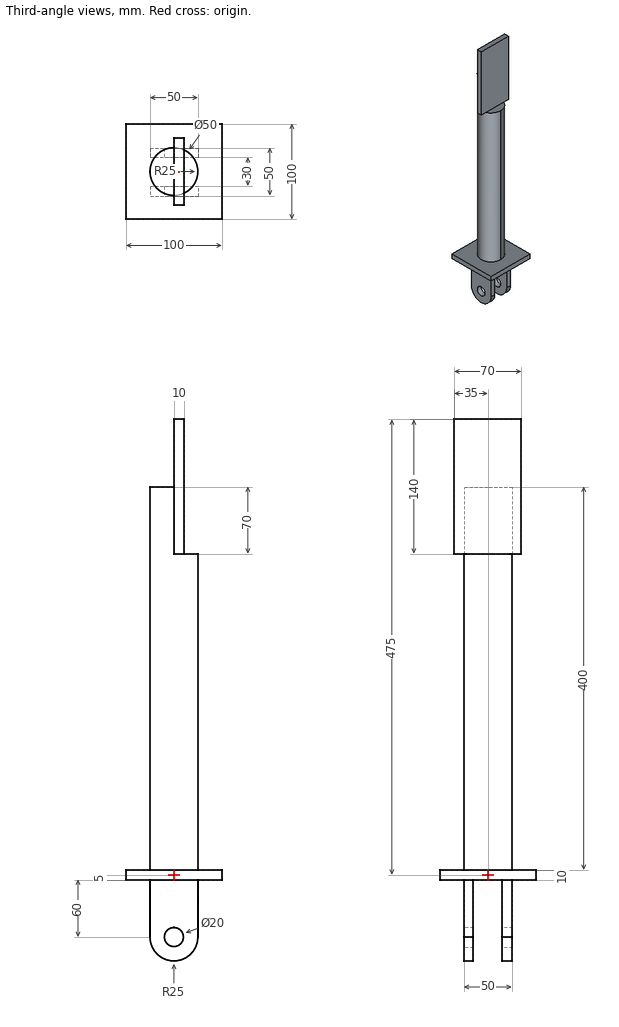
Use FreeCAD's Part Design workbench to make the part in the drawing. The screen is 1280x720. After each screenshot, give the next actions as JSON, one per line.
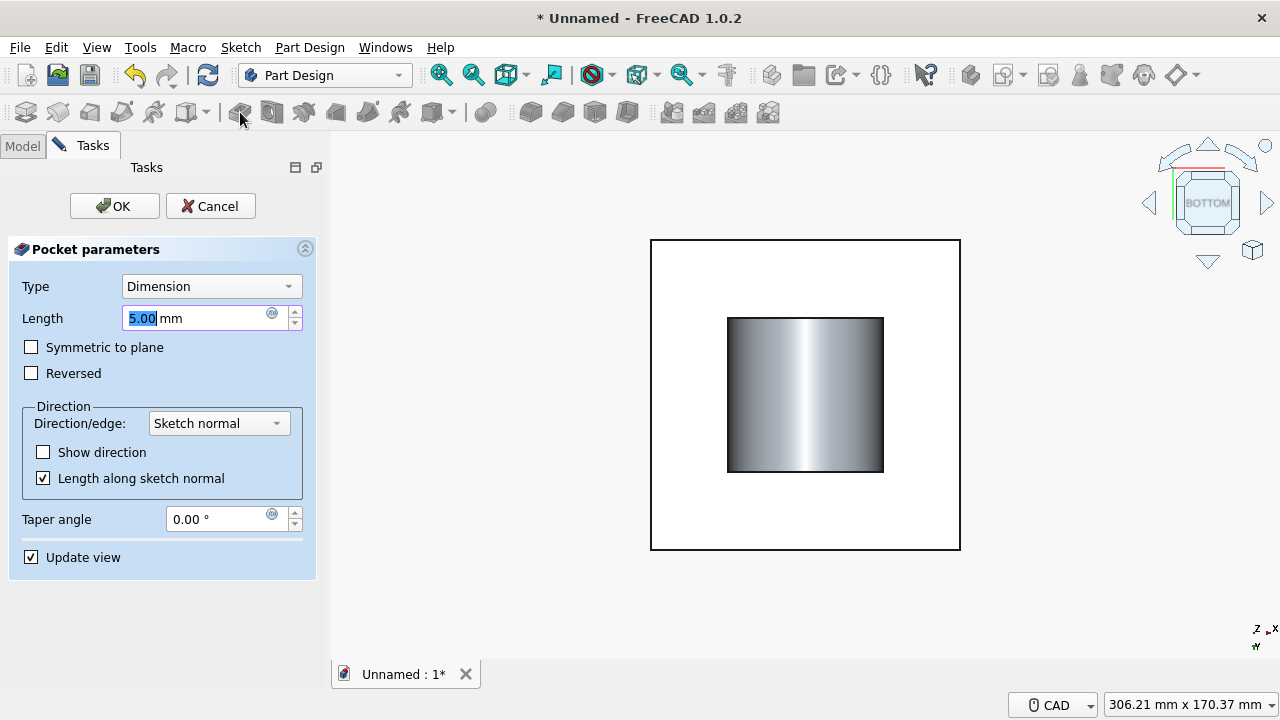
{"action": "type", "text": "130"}
{"action": "key", "text": "Tab"}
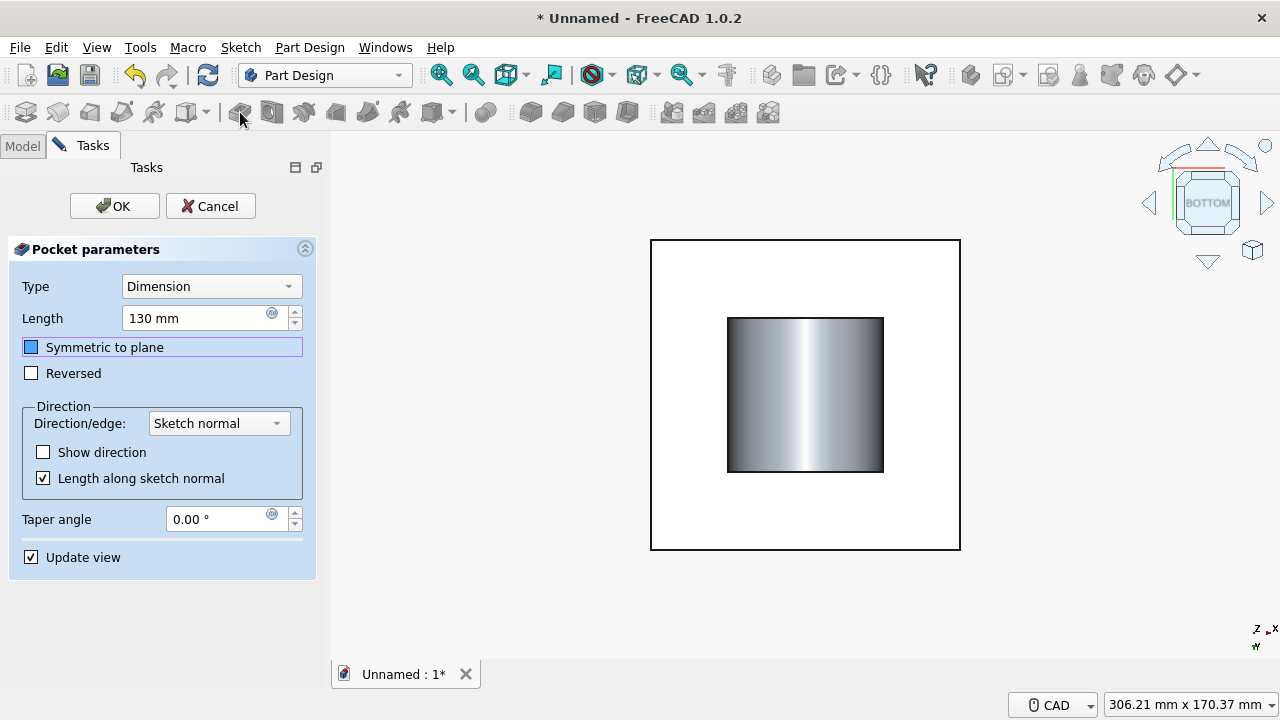
{"action": "left_click", "coordinate": [30, 373]}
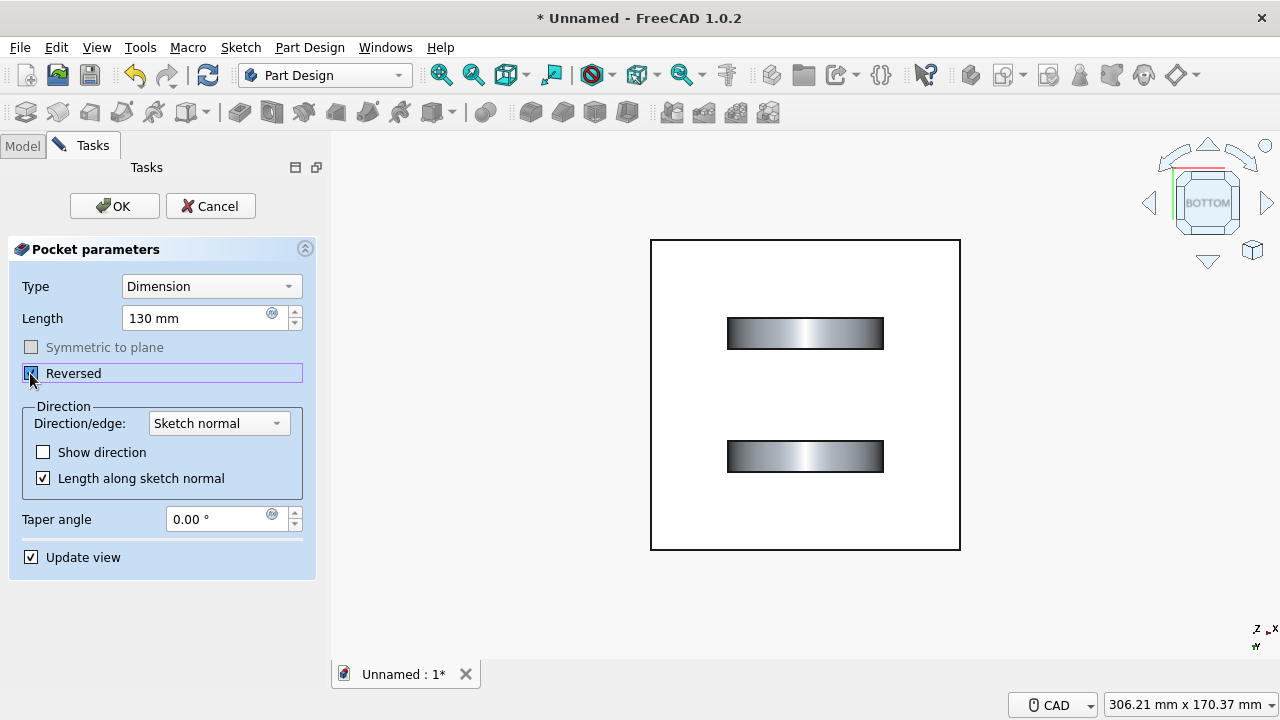
{"action": "left_click", "coordinate": [115, 206]}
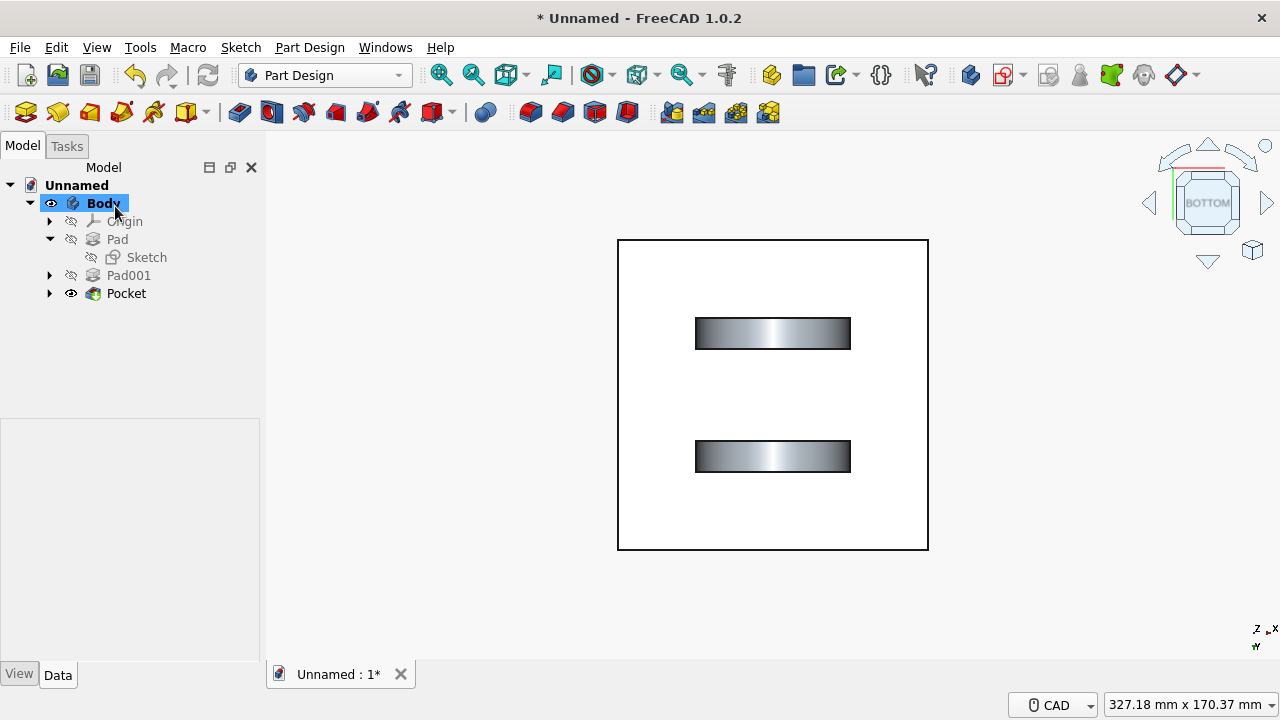
{"action": "key", "text": "0"}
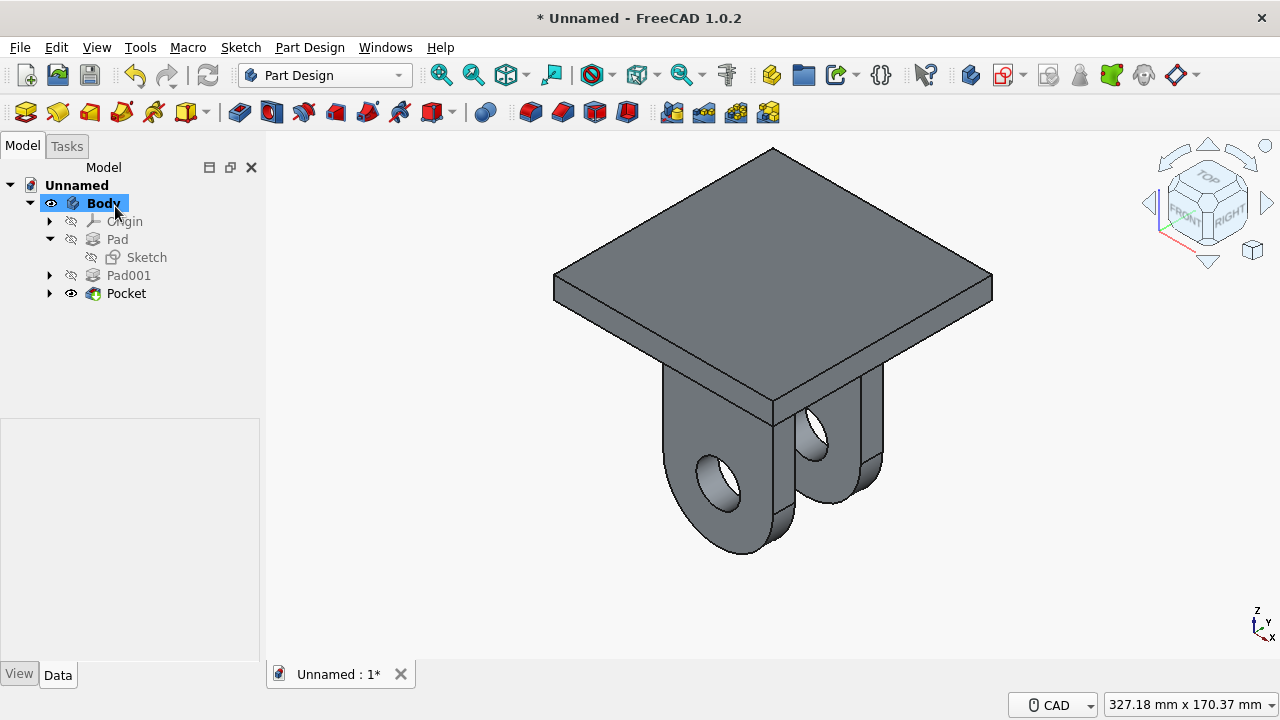
{"action": "left_click", "coordinate": [773, 274]}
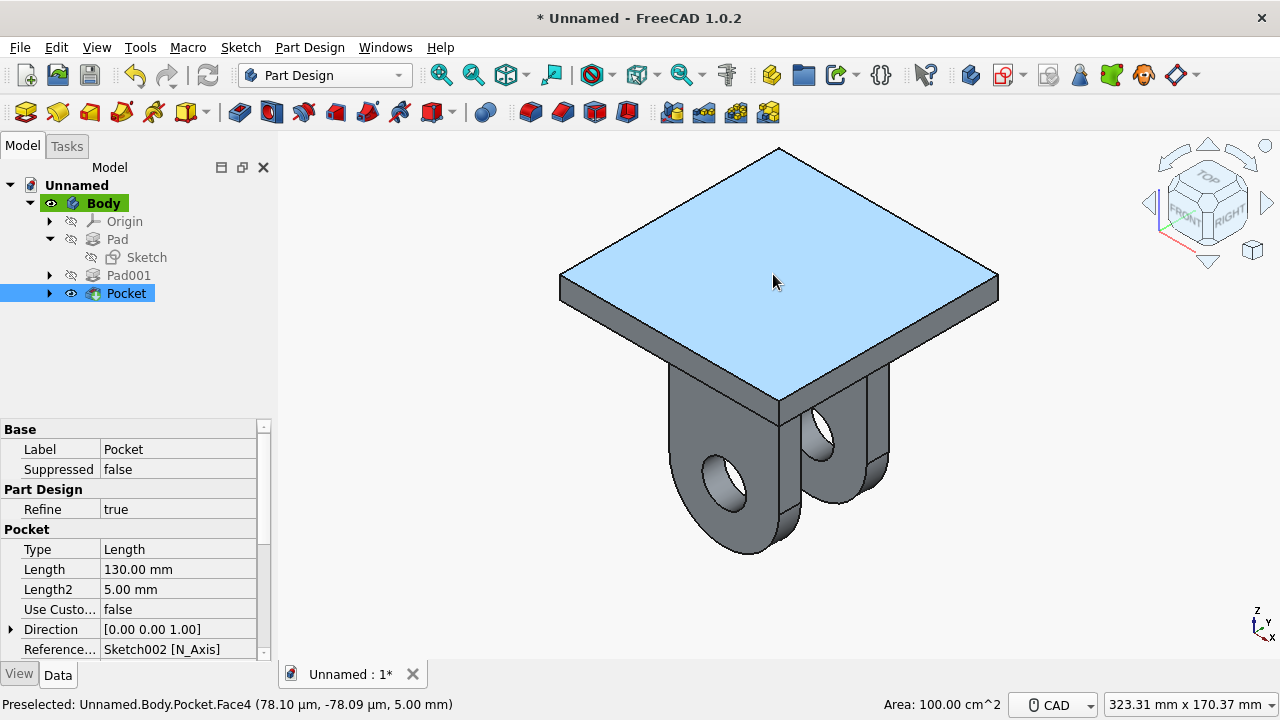
{"action": "left_click", "coordinate": [1004, 76]}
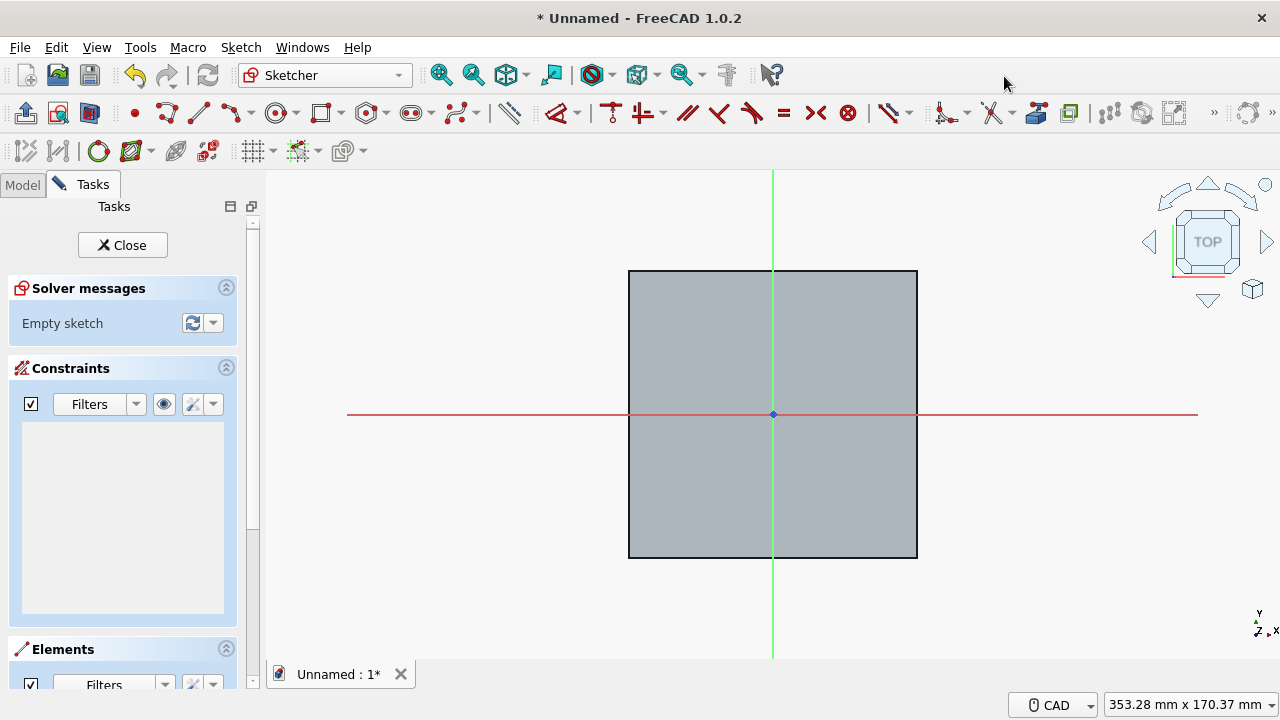
{"action": "scroll", "coordinate": [829, 414], "scroll_direction": "up", "scroll_amount": 4}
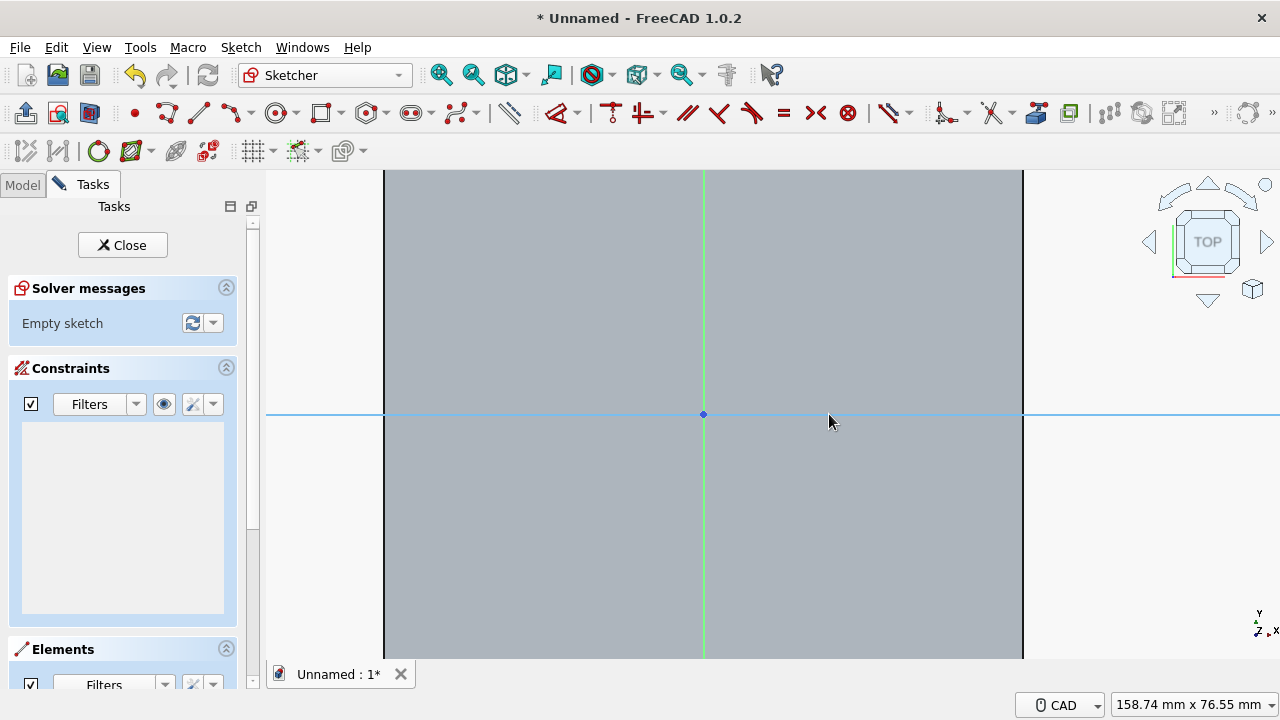
{"action": "key", "text": "g c"}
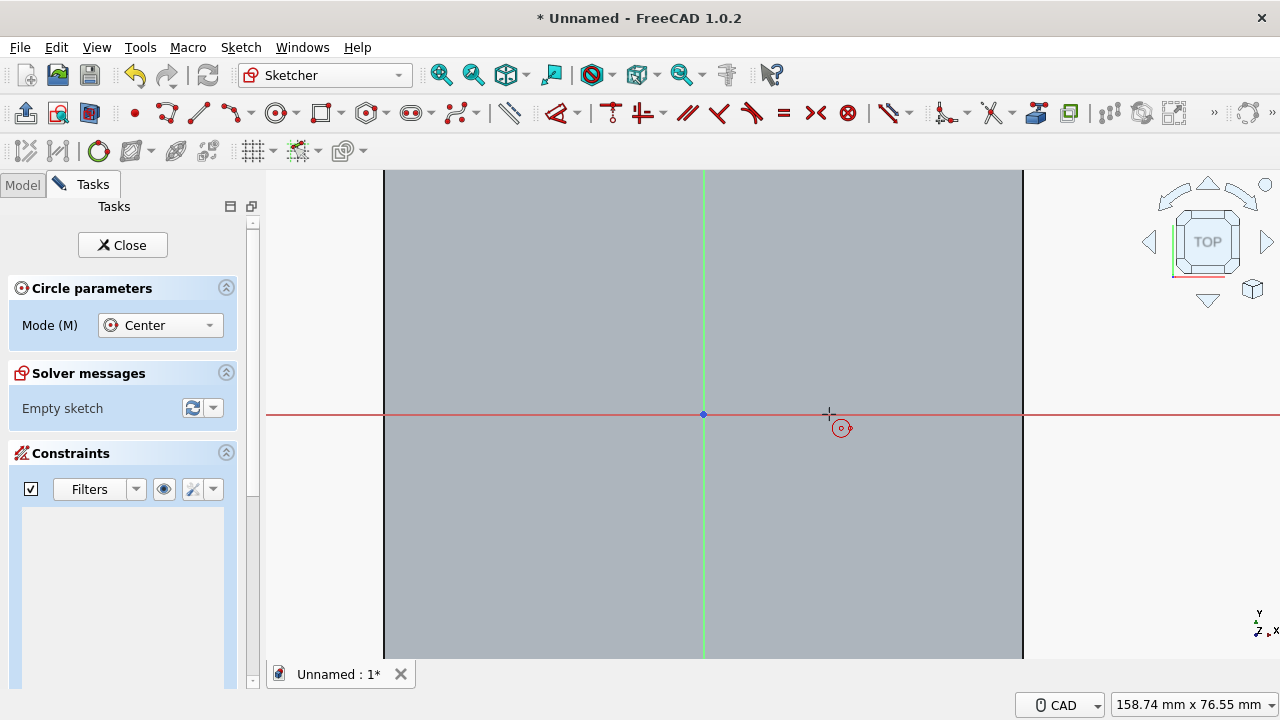
{"action": "left_click", "coordinate": [704, 414]}
{"action": "left_click", "coordinate": [817, 302]}
{"action": "key", "text": "Escape"}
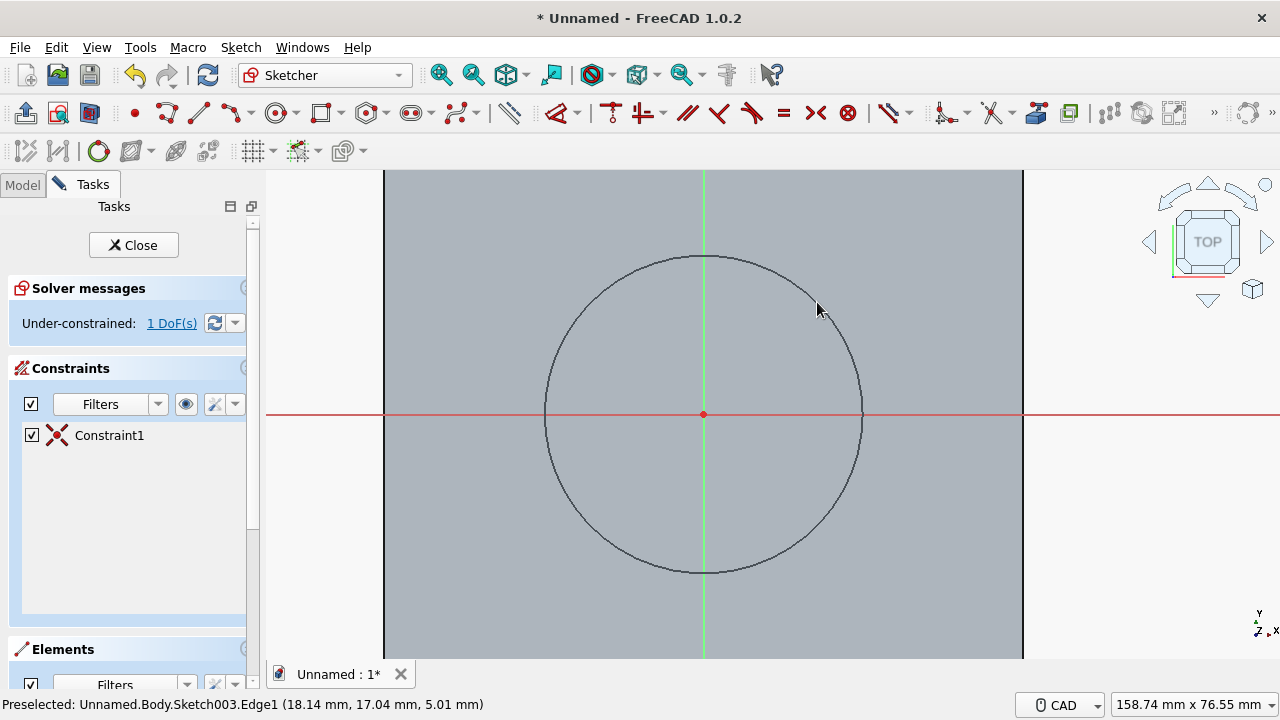
{"action": "key", "text": "d"}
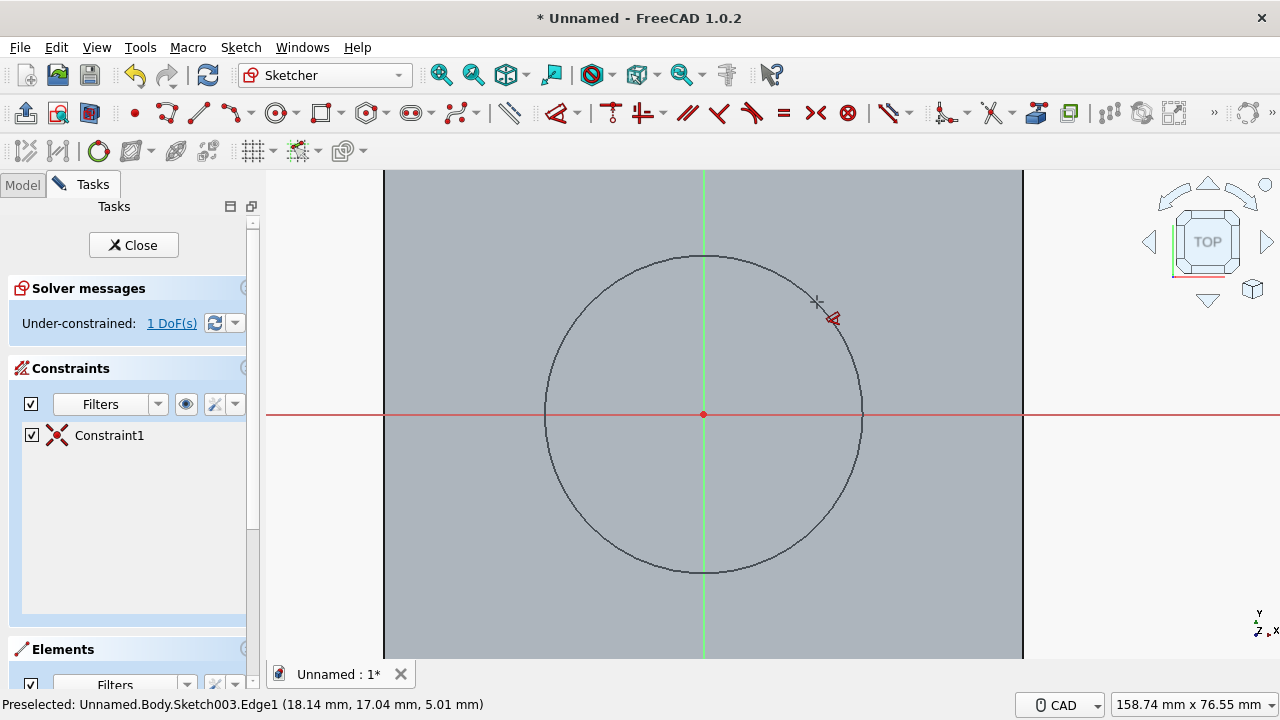
{"action": "left_click", "coordinate": [816, 302]}
{"action": "left_click", "coordinate": [839, 279]}